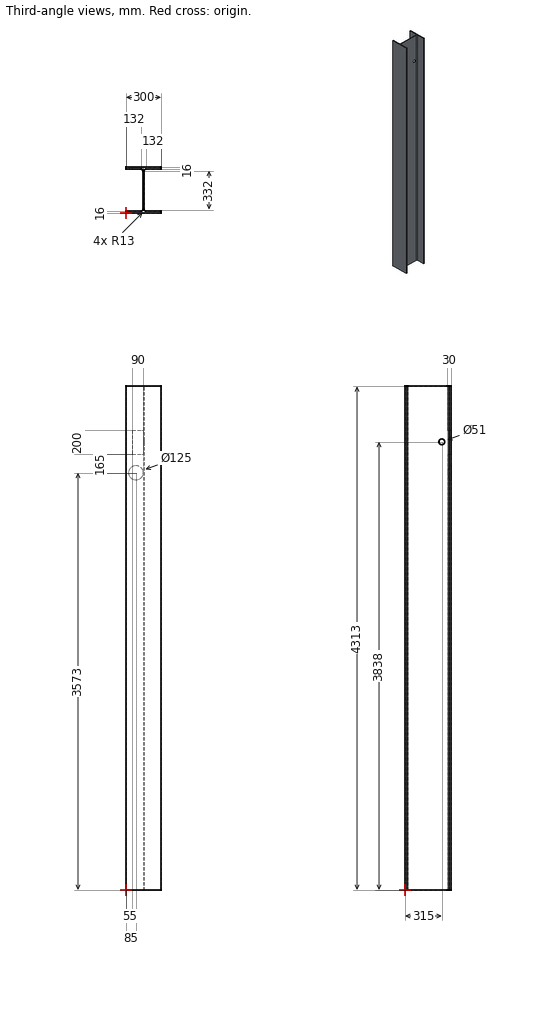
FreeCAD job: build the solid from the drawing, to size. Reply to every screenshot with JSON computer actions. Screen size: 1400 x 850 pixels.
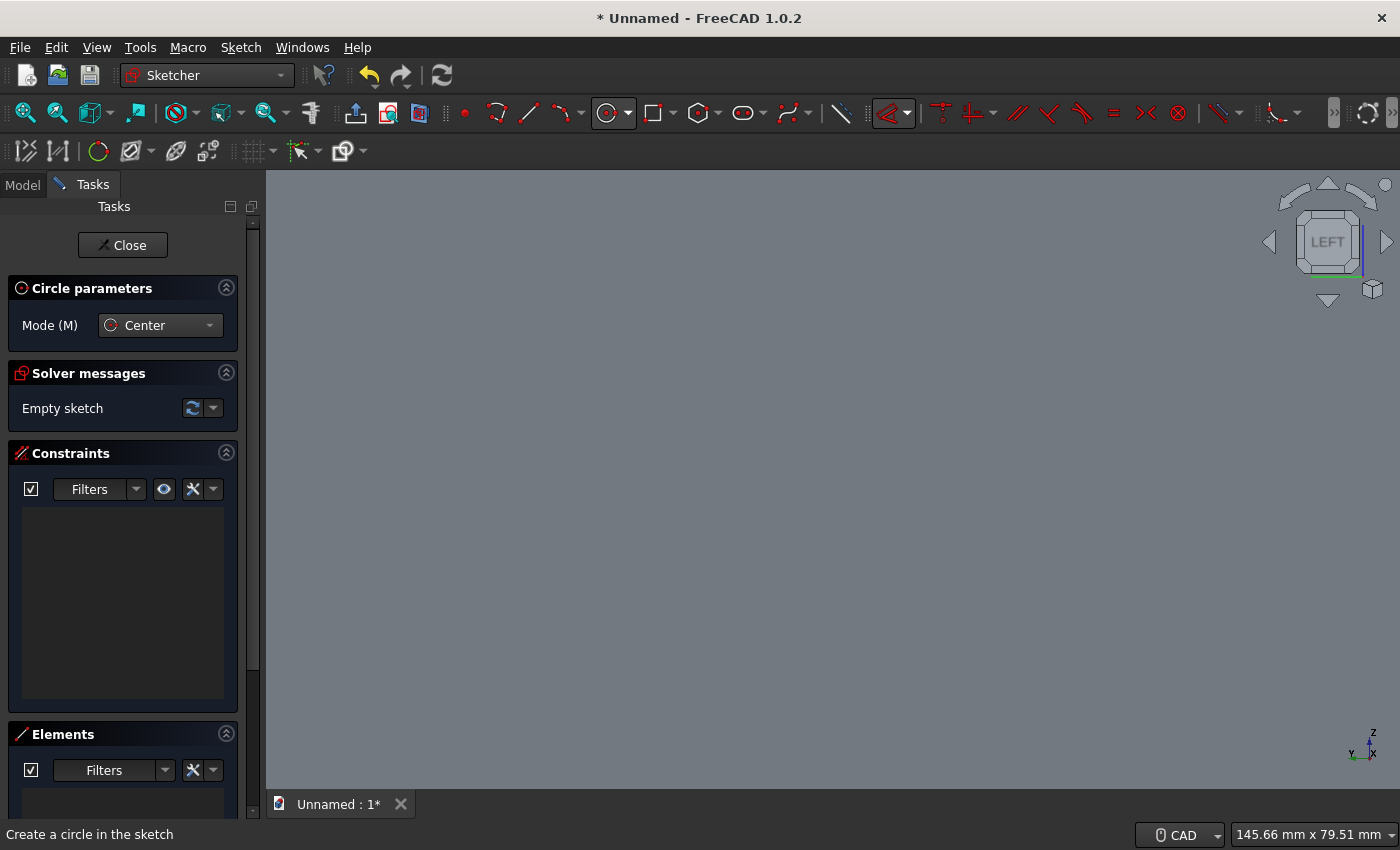
{"action": "left_click", "coordinate": [765, 479]}
{"action": "mouse_move", "coordinate": [905, 339]}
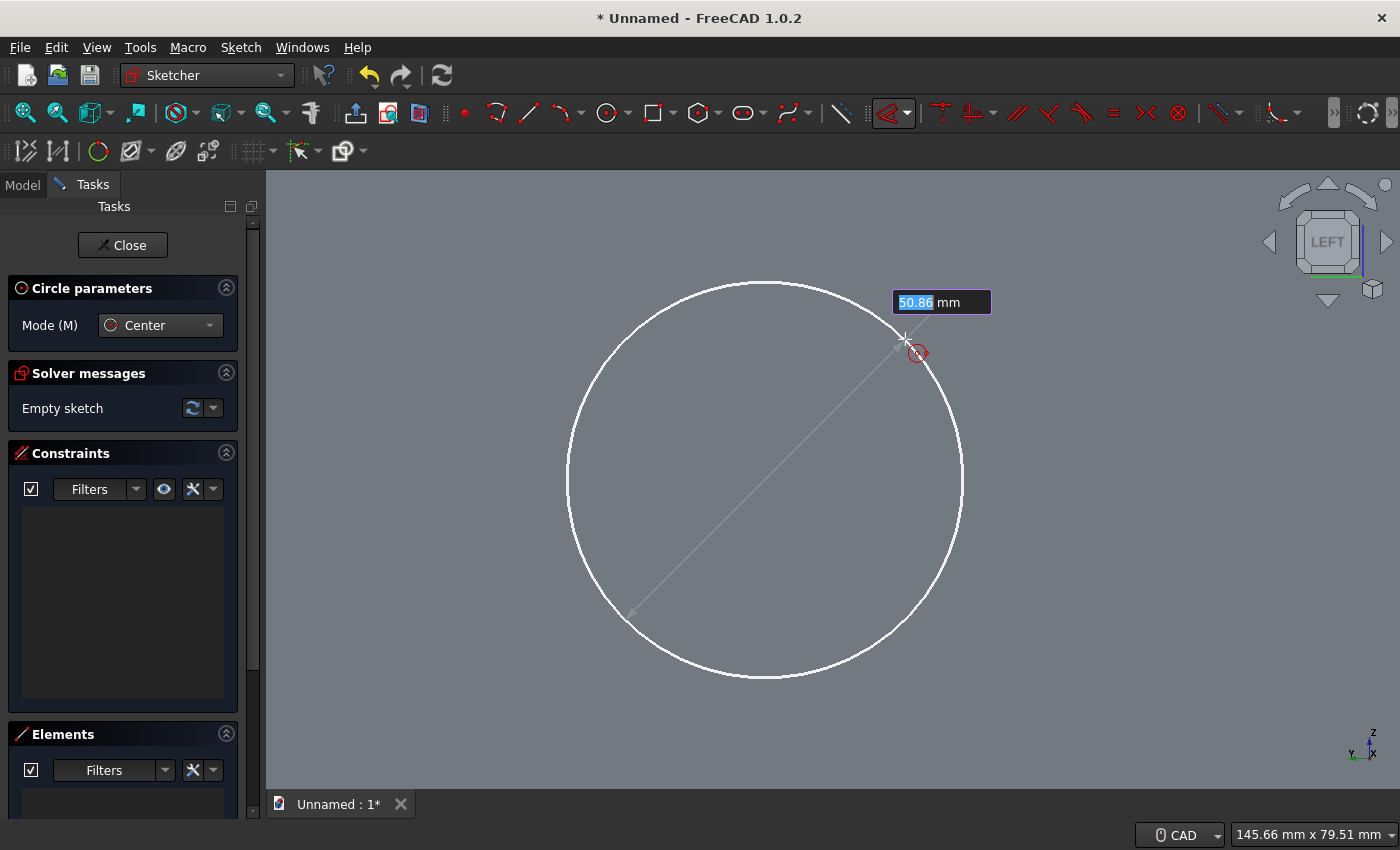
{"action": "type", "text": "51"}
{"action": "key", "text": "Return"}
{"action": "key", "text": "Escape"}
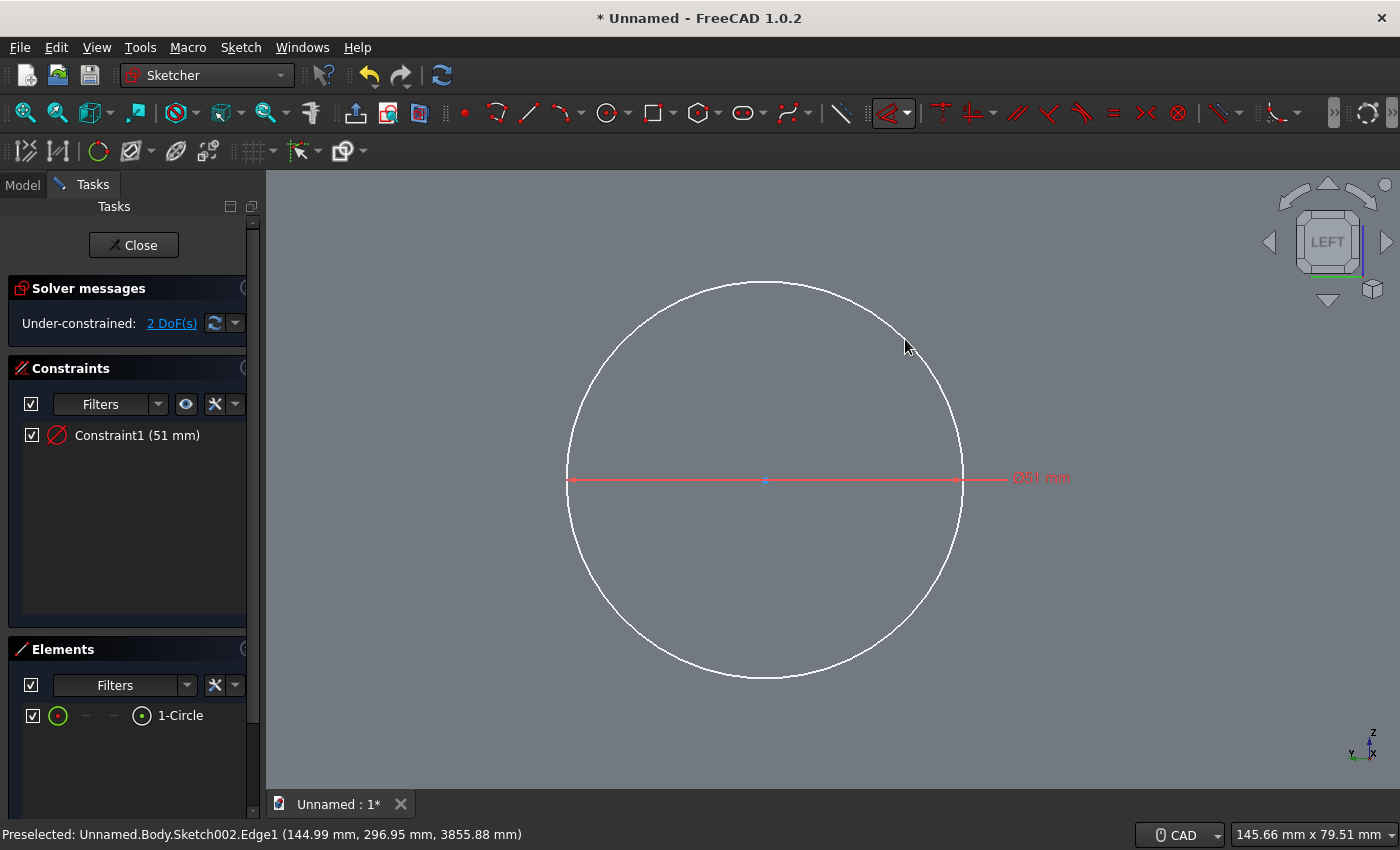
{"action": "left_click", "coordinate": [765, 480]}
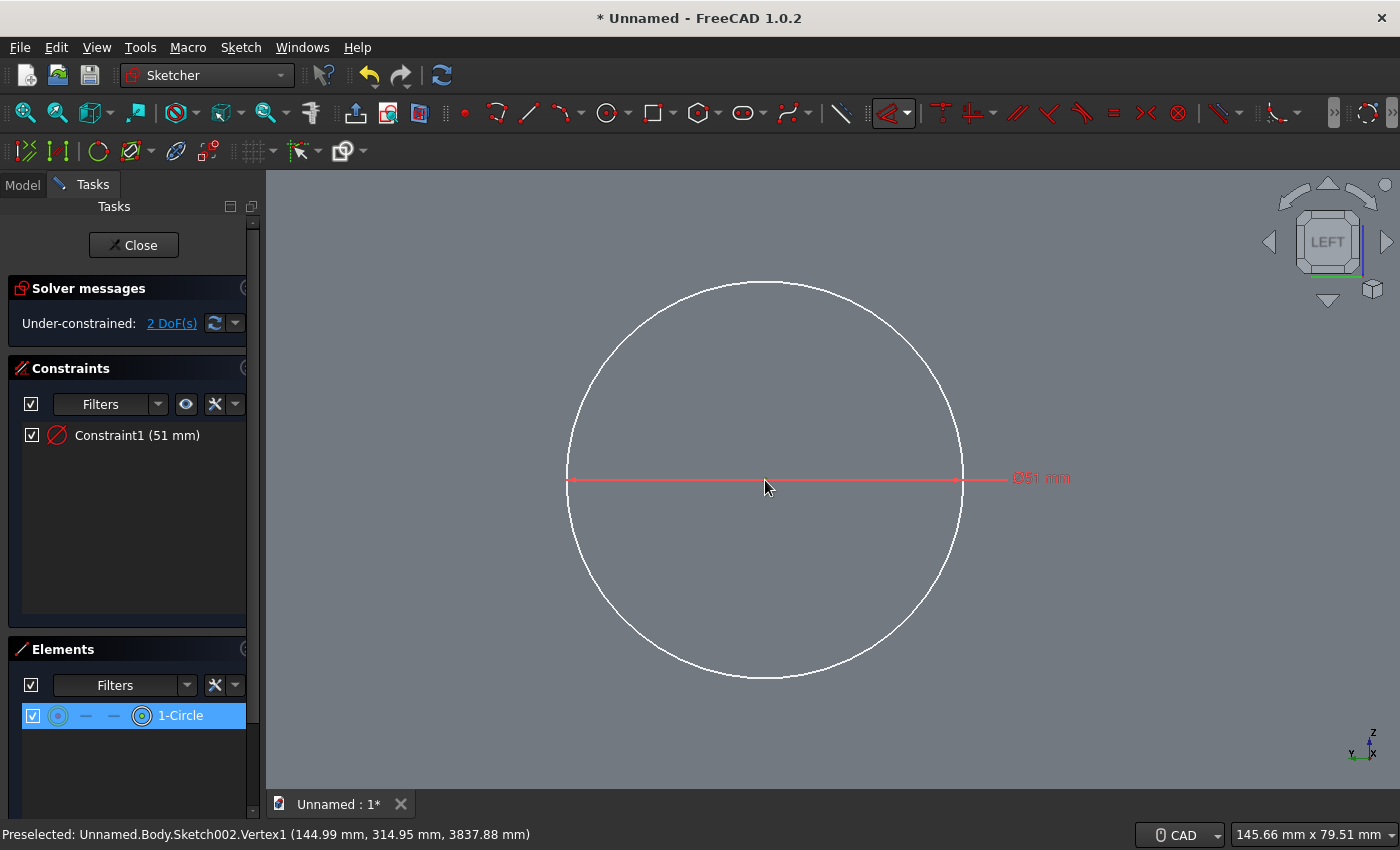
{"action": "left_click", "coordinate": [910, 114]}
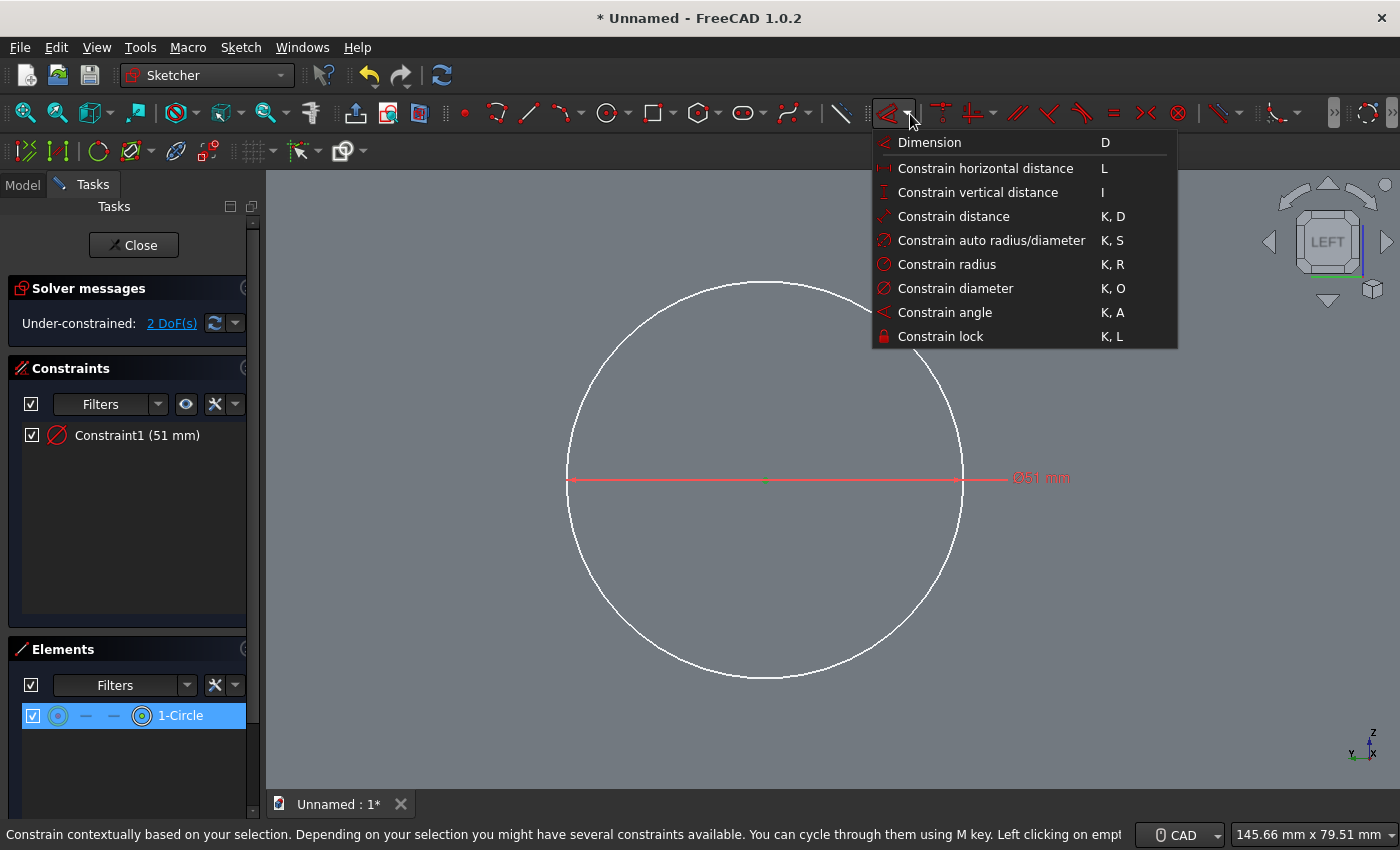
{"action": "left_click", "coordinate": [1025, 168]}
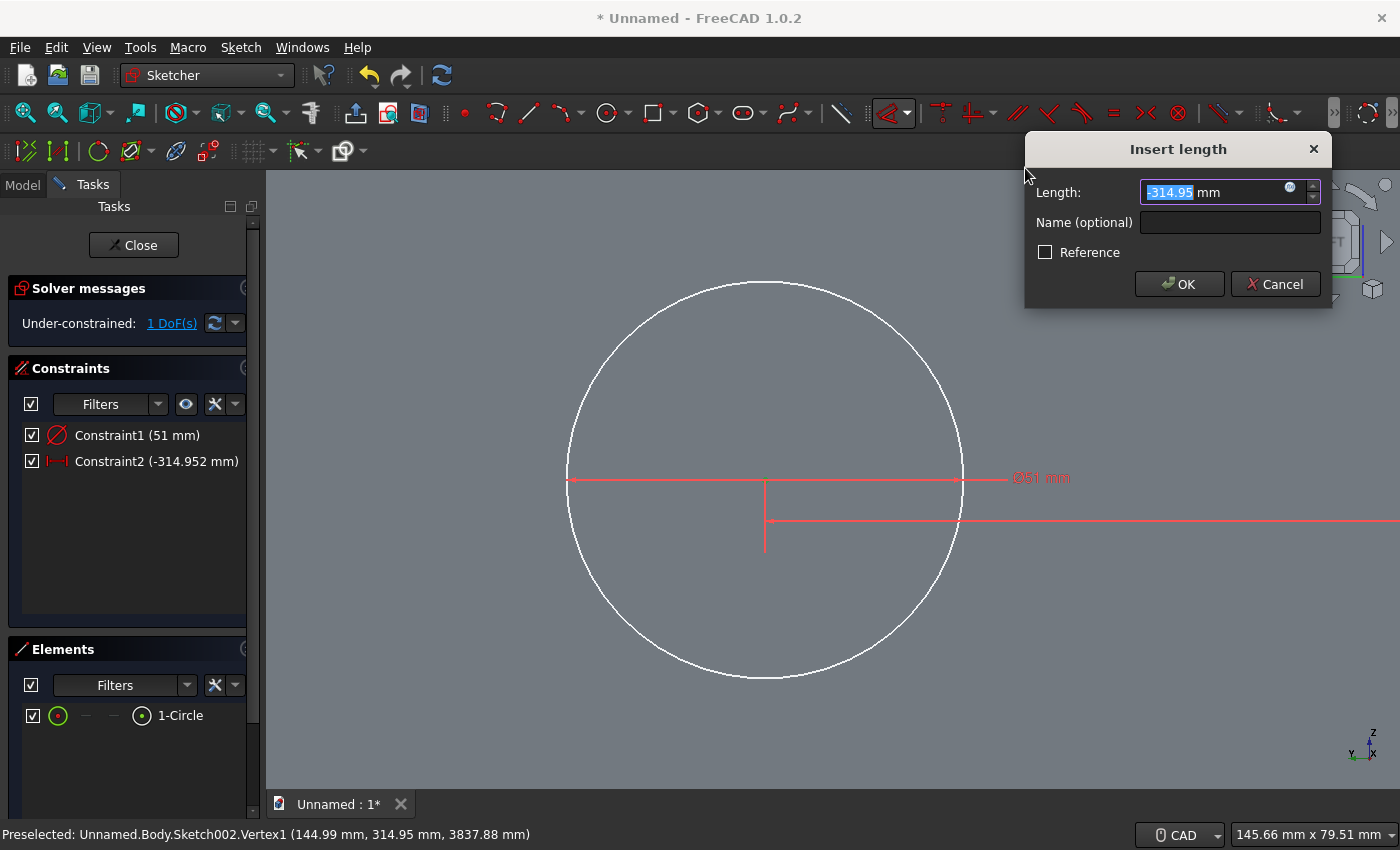
{"action": "type", "text": "-315"}
{"action": "key", "text": "Return"}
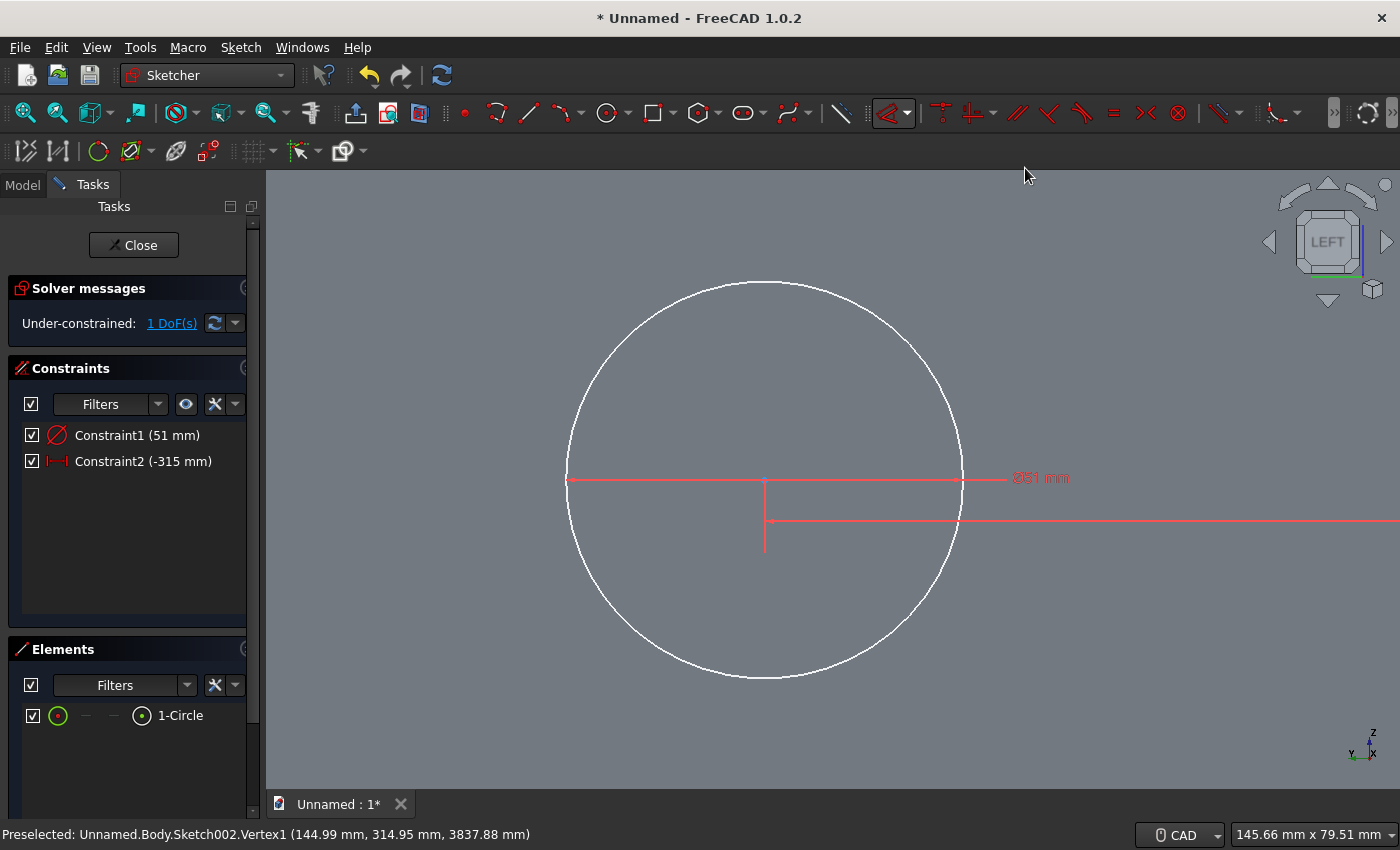
{"action": "left_click", "coordinate": [765, 480]}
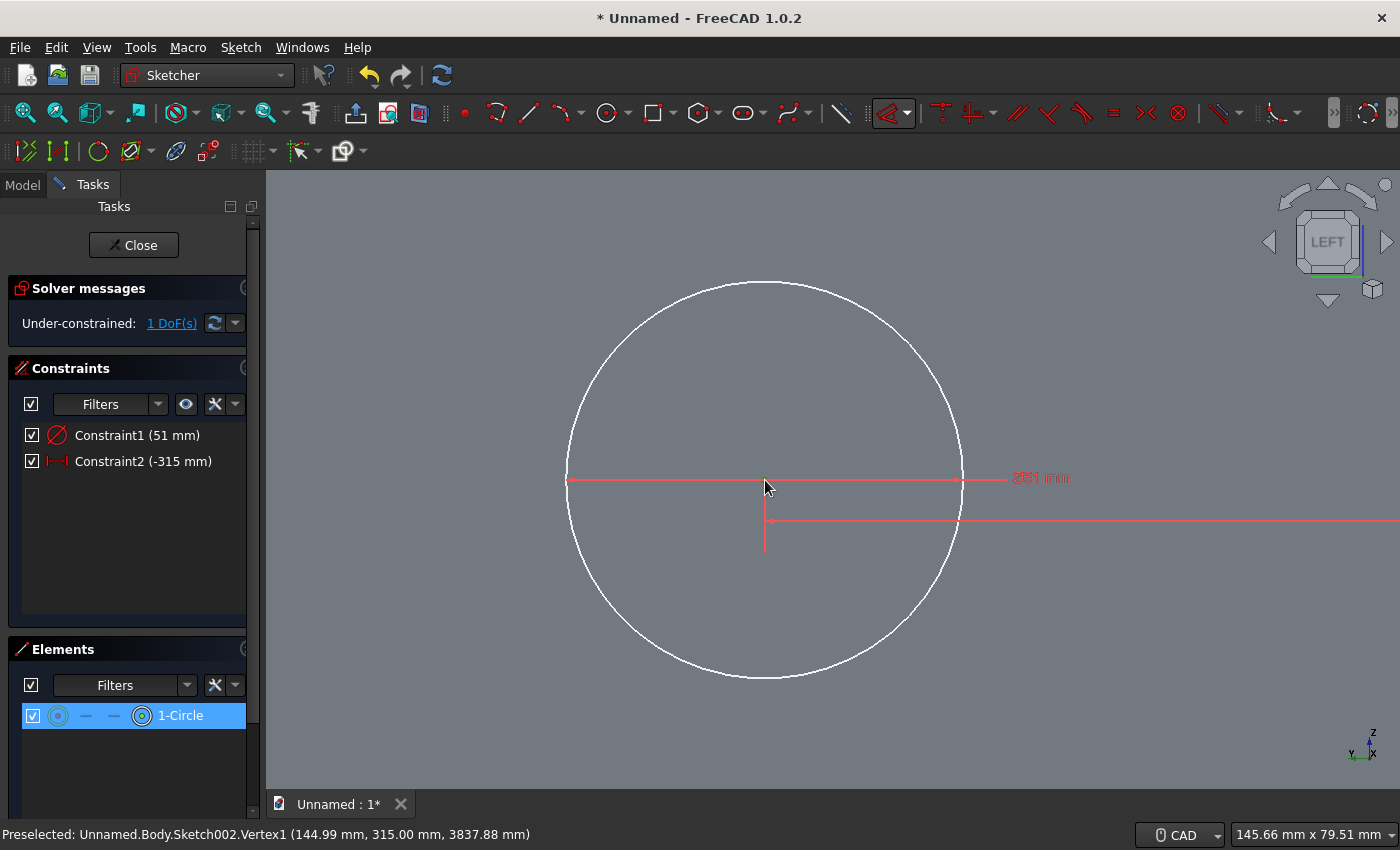
{"action": "key", "text": "i"}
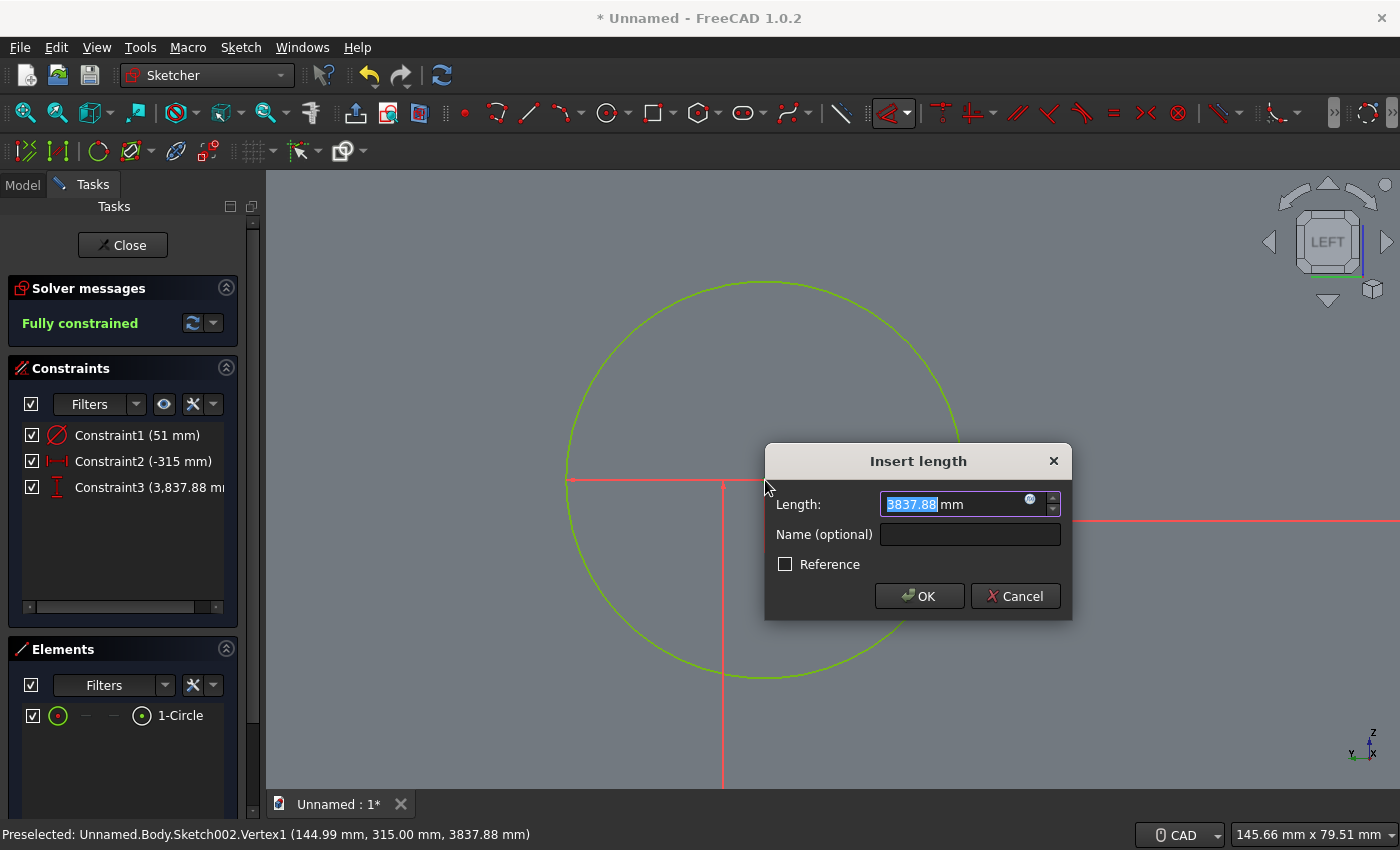
{"action": "type", "text": "3838"}
{"action": "key", "text": "Return"}